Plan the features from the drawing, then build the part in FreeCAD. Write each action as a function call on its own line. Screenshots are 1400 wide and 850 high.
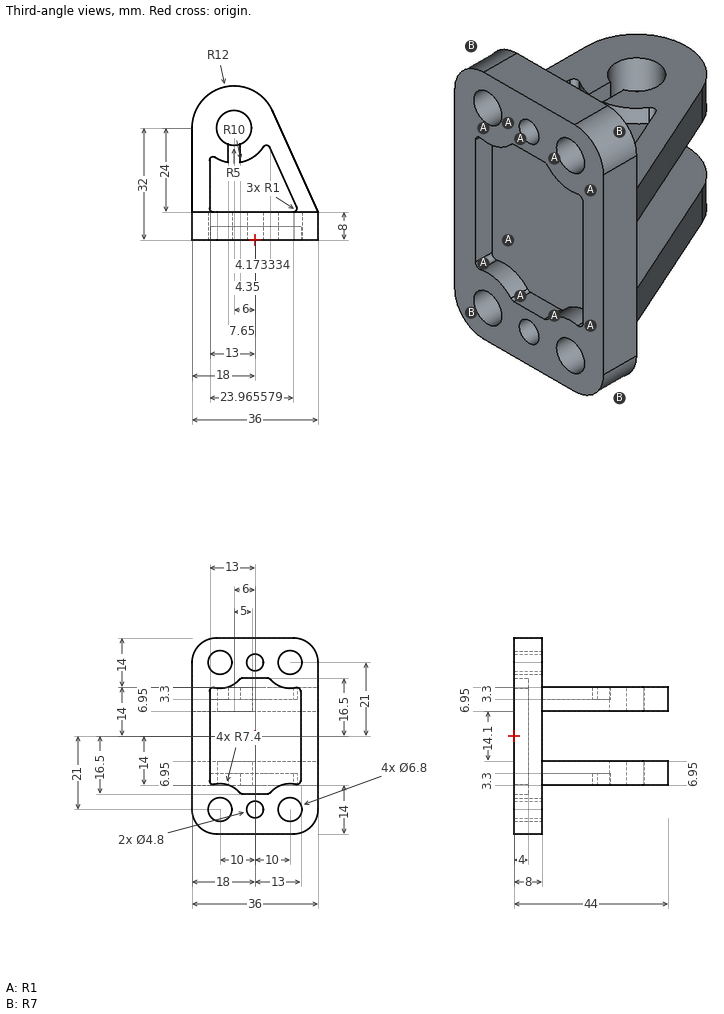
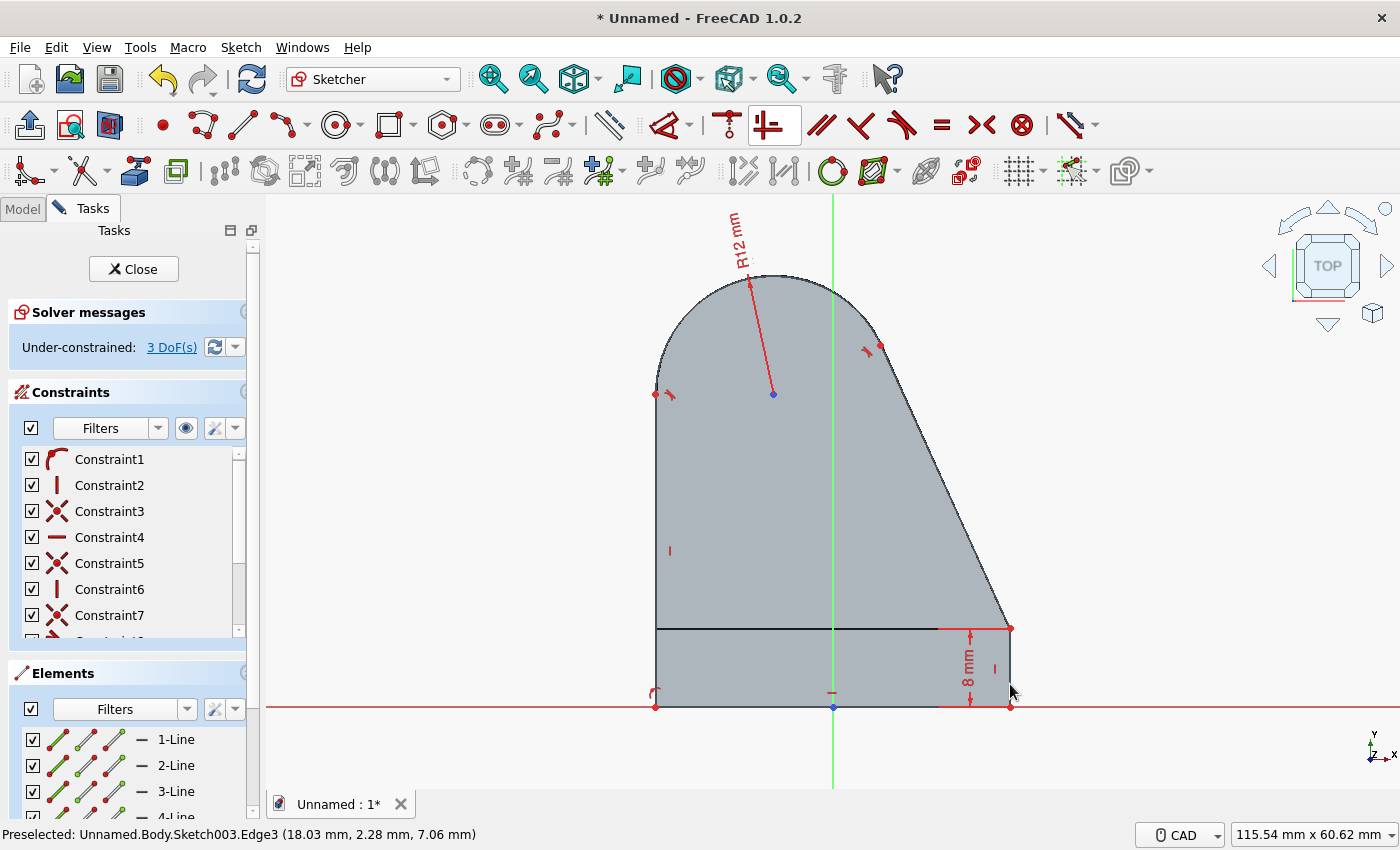
click(656, 488)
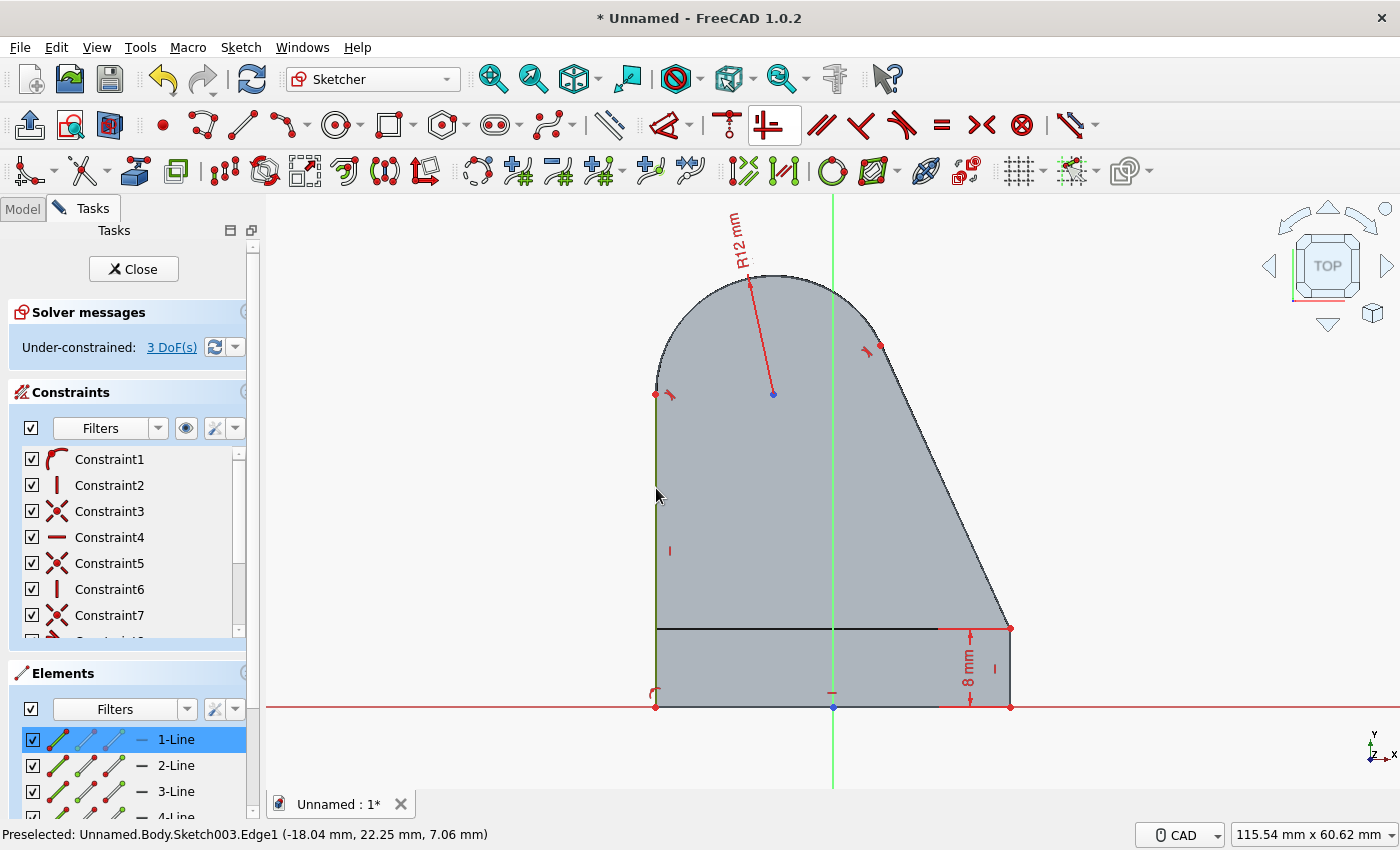
key(i)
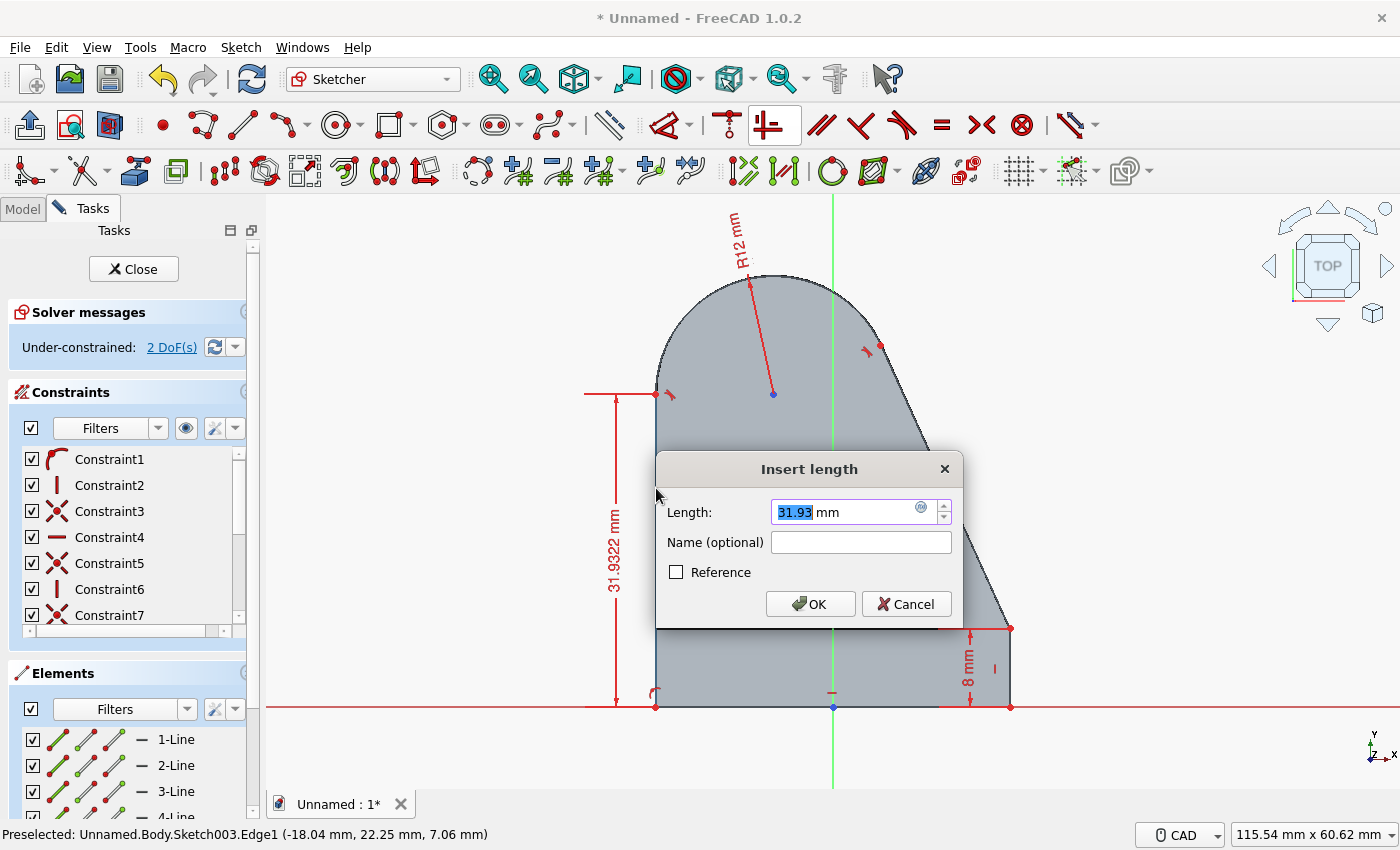
text(32)
key(Return)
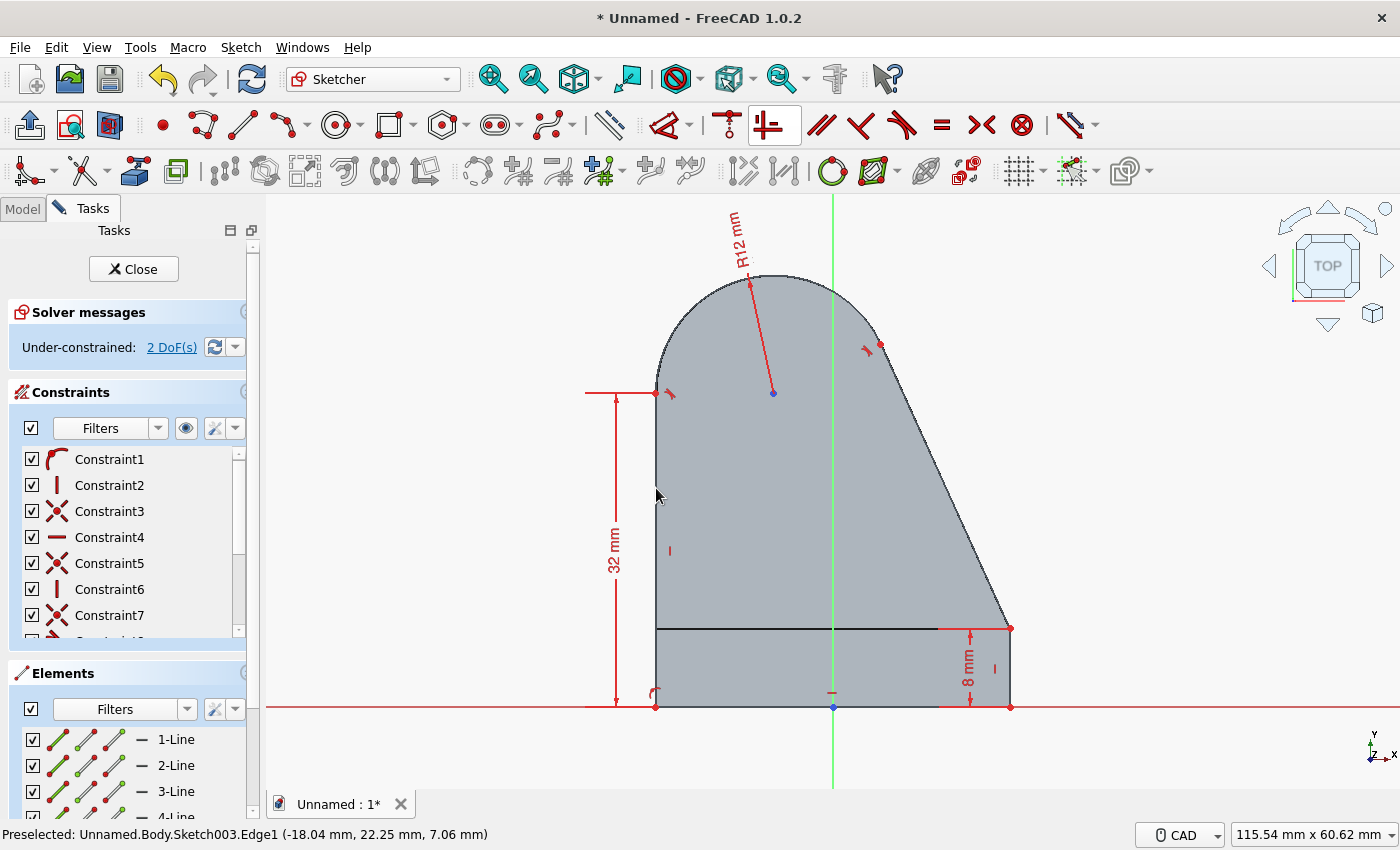
click(762, 707)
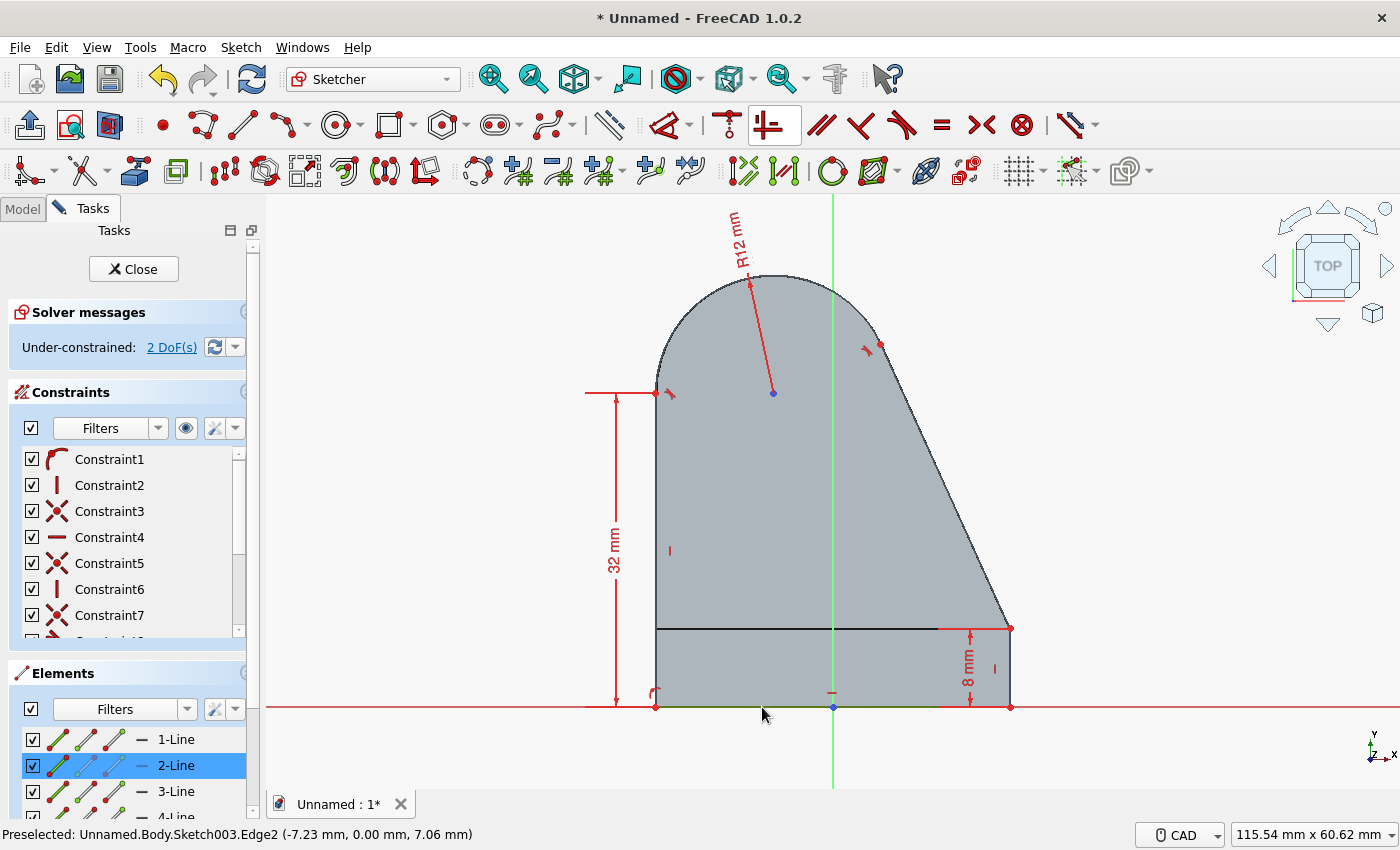
click(692, 126)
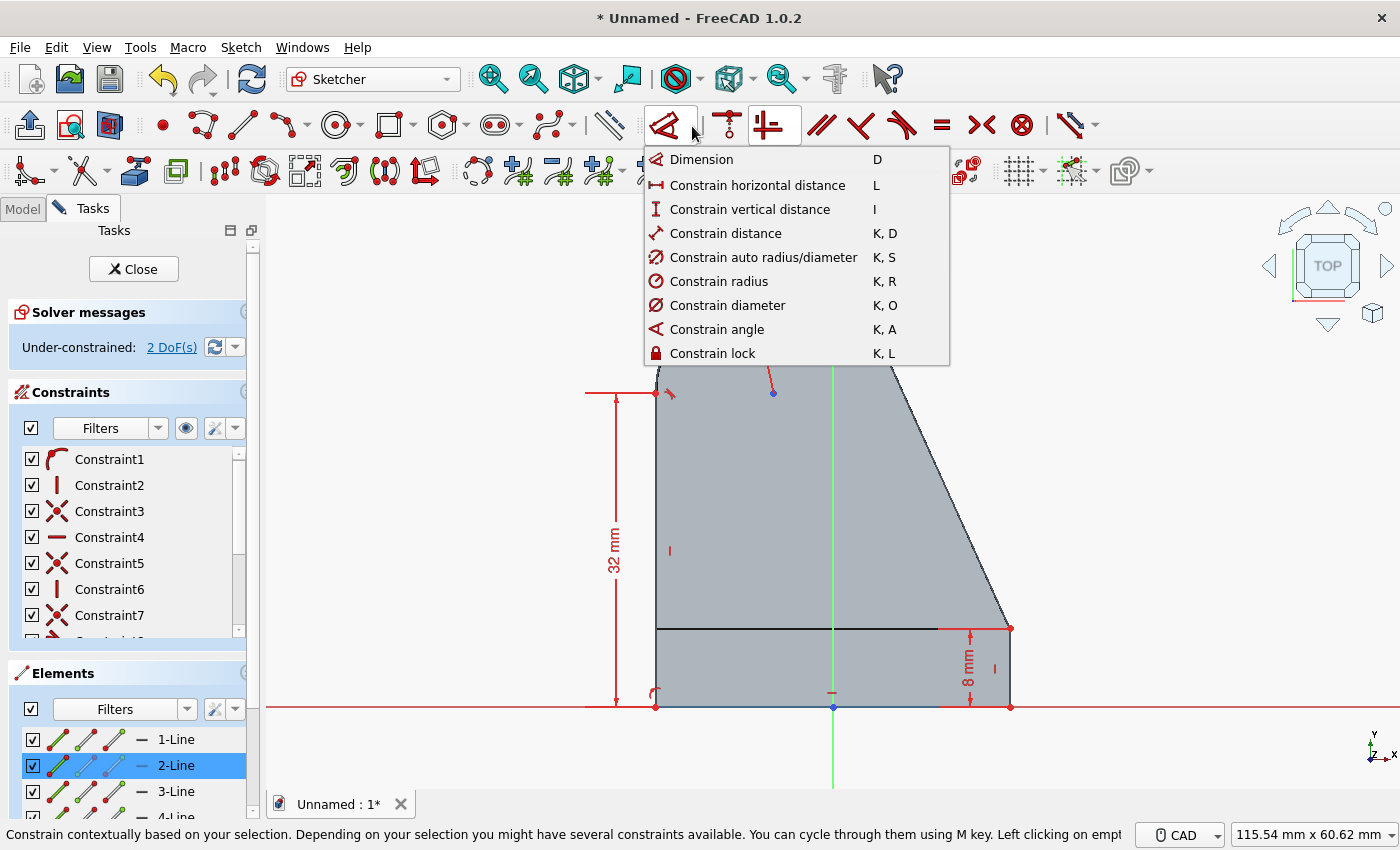
click(797, 185)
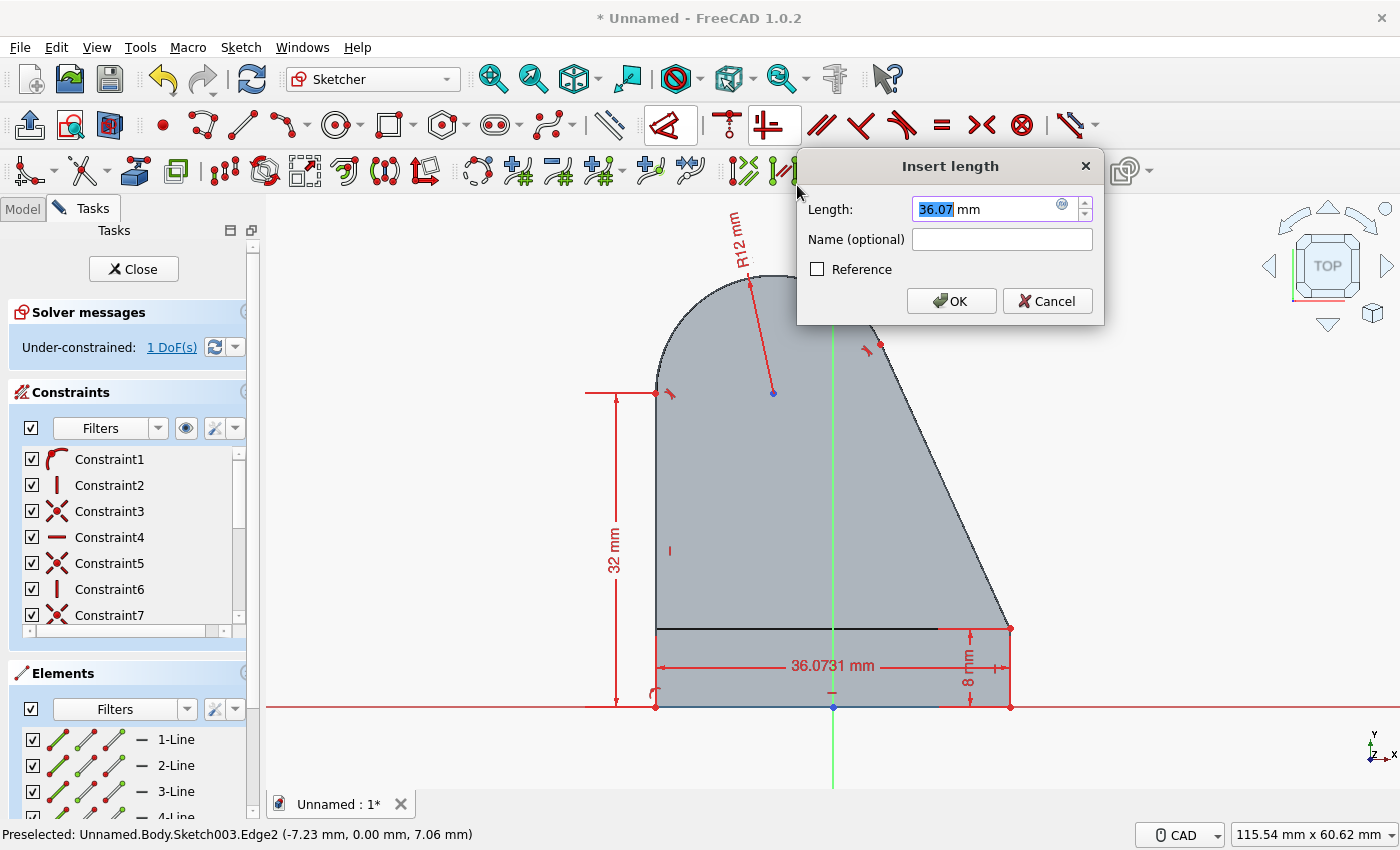
text(36)
key(Return)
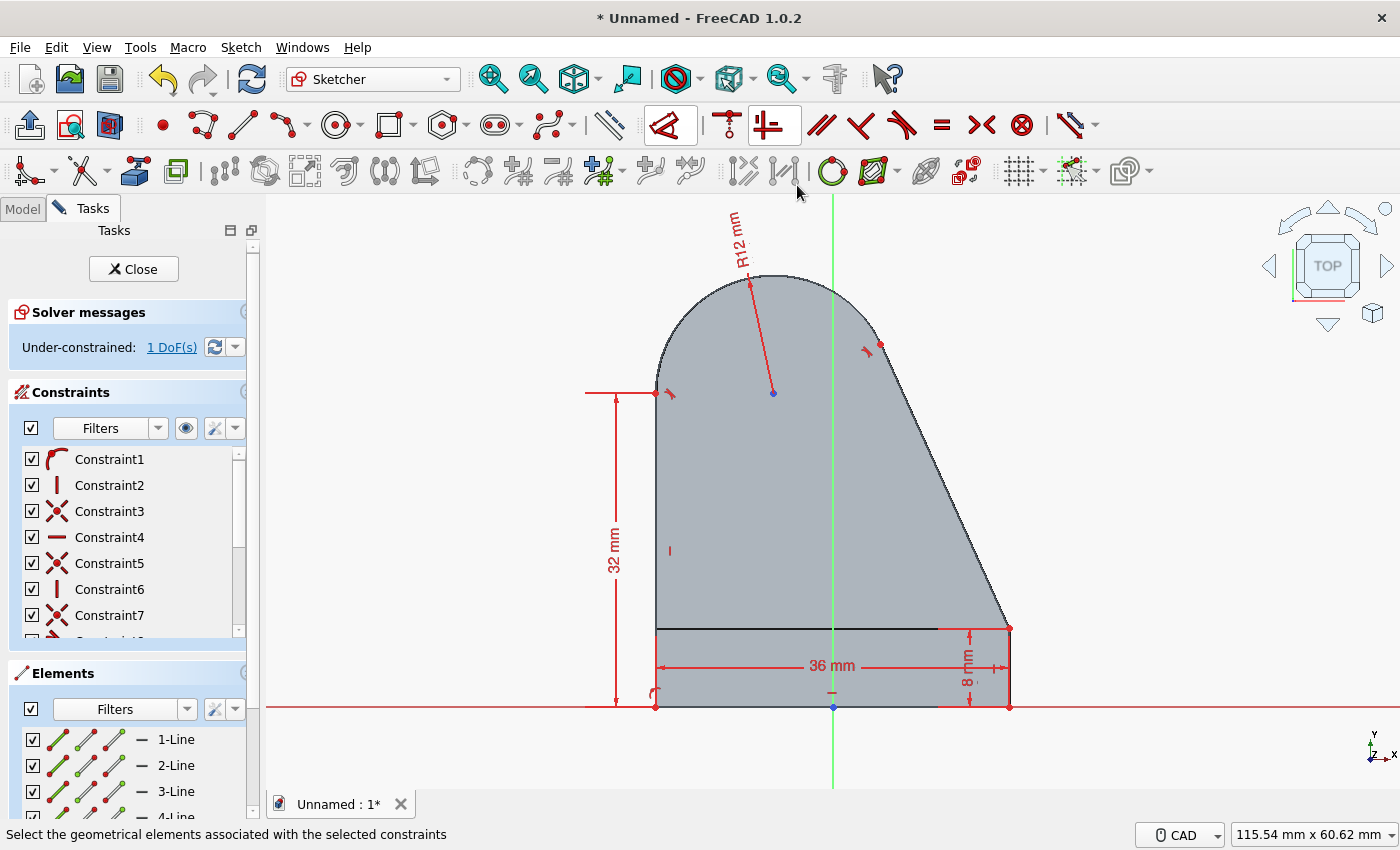
click(774, 393)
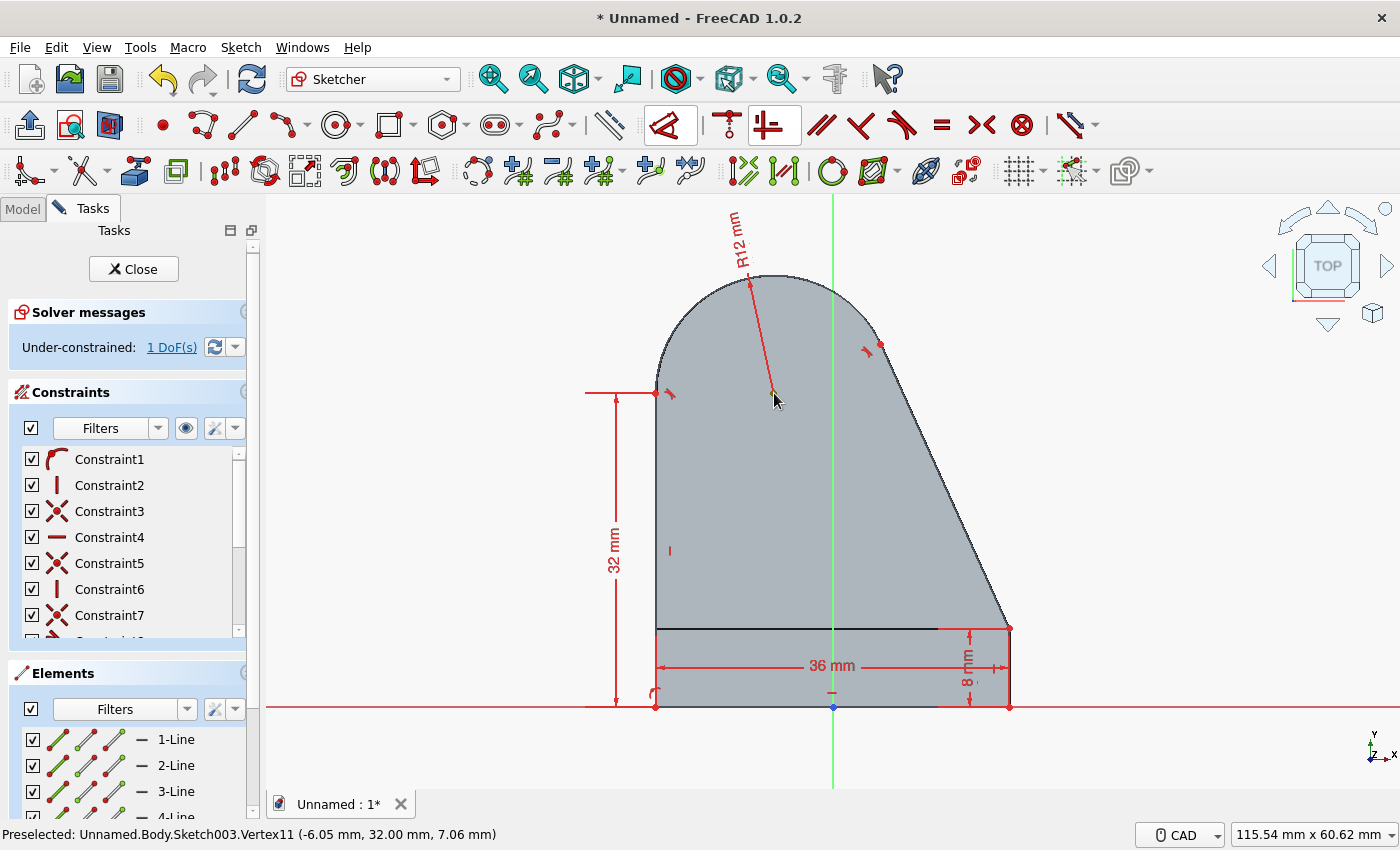
key(l)